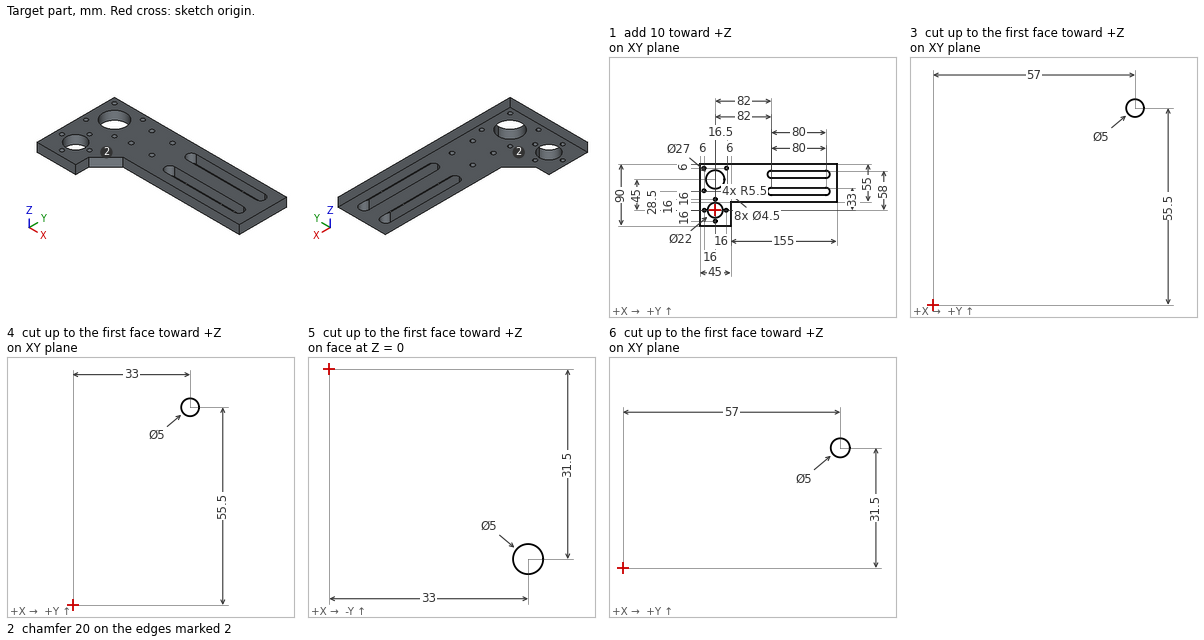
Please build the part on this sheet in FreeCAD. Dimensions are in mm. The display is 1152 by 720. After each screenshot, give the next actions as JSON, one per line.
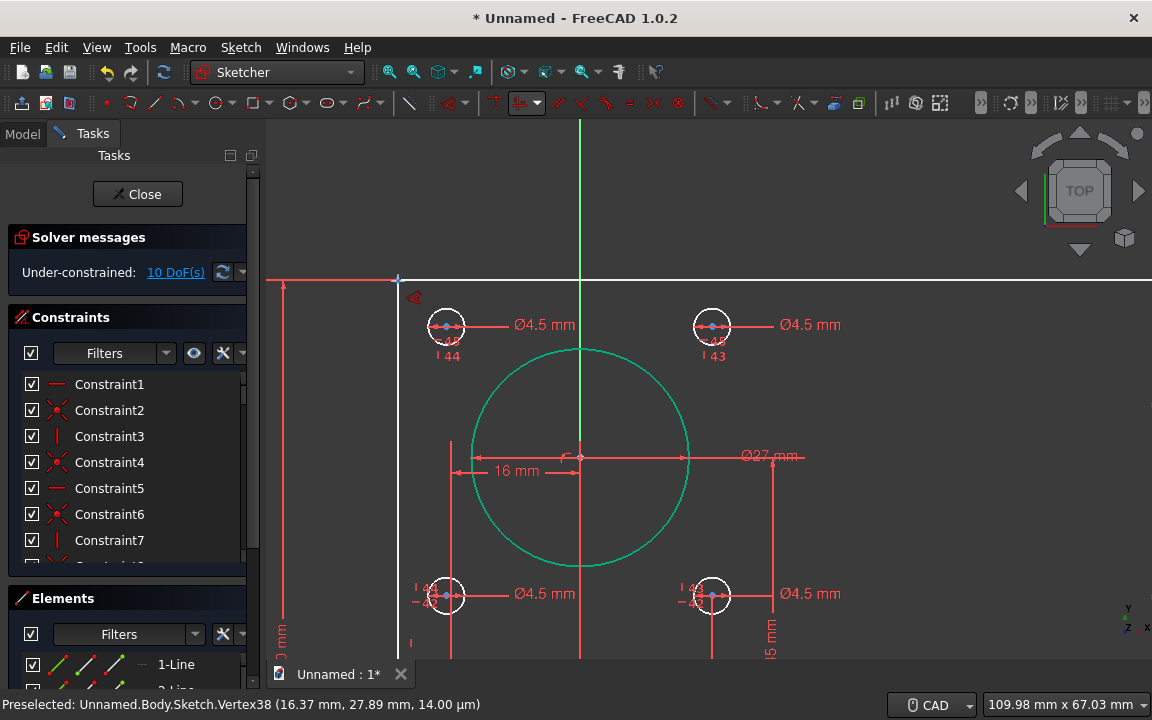
{"action": "left_click", "coordinate": [398, 280]}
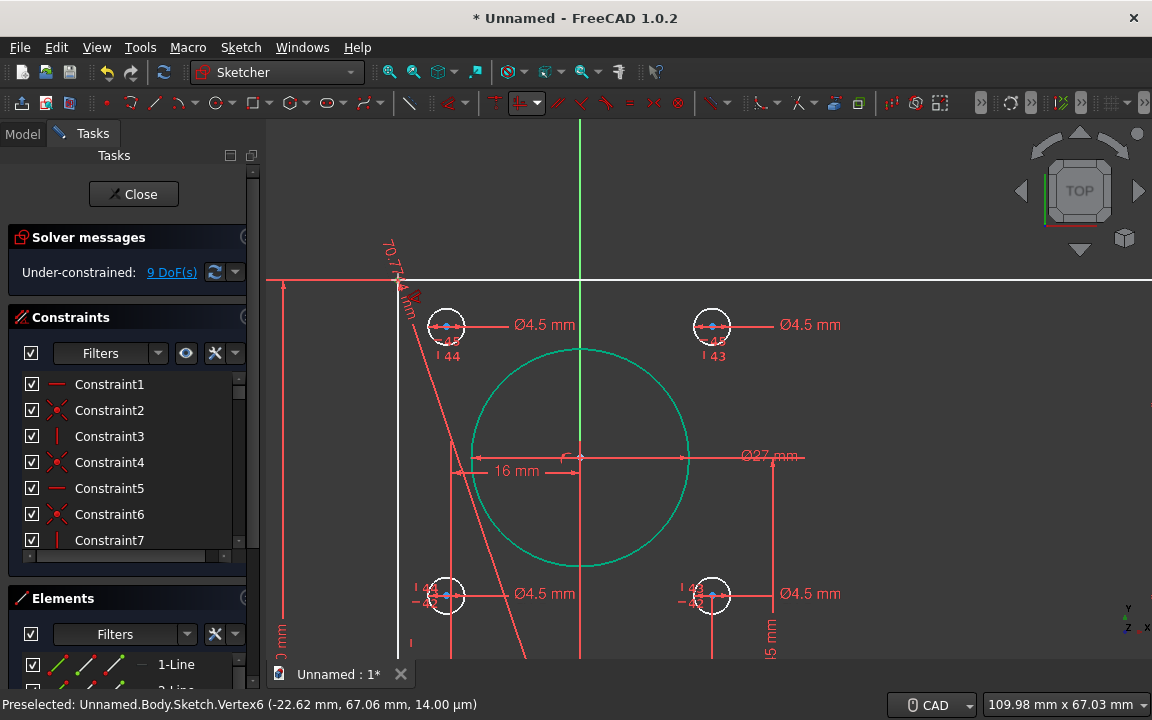
{"action": "left_click", "coordinate": [446, 596]}
{"action": "left_click", "coordinate": [422, 246]}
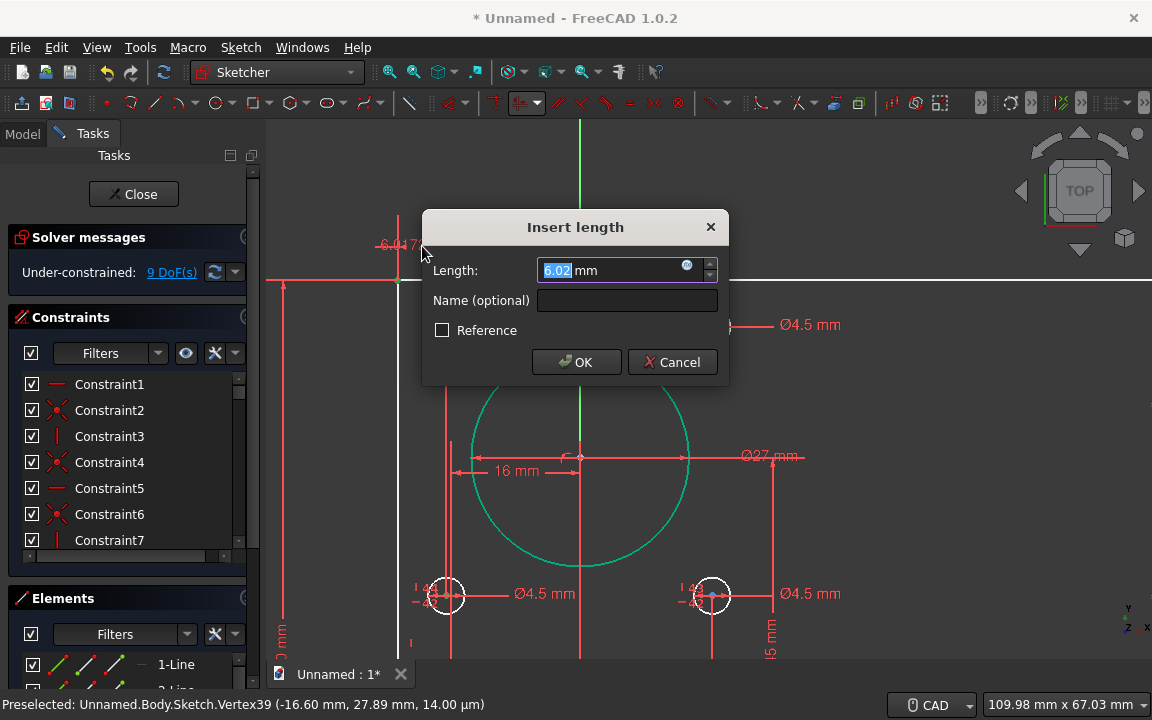
{"action": "type", "text": "6"}
{"action": "key", "text": "Return"}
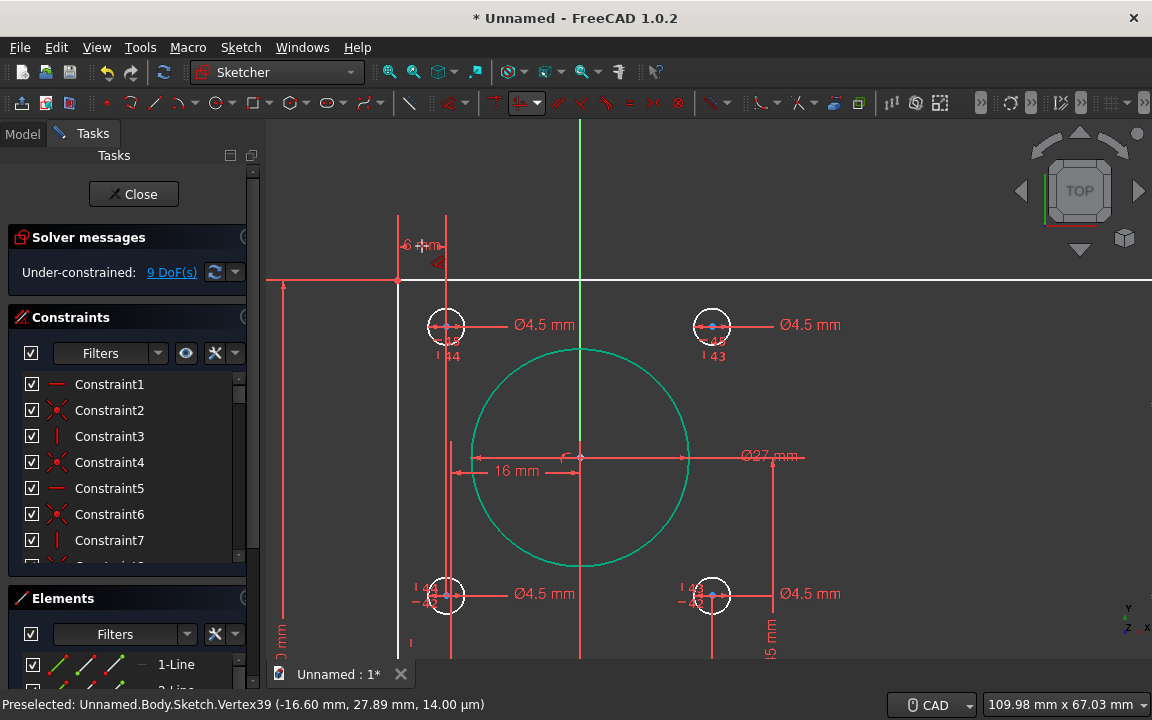
{"action": "left_click", "coordinate": [398, 280]}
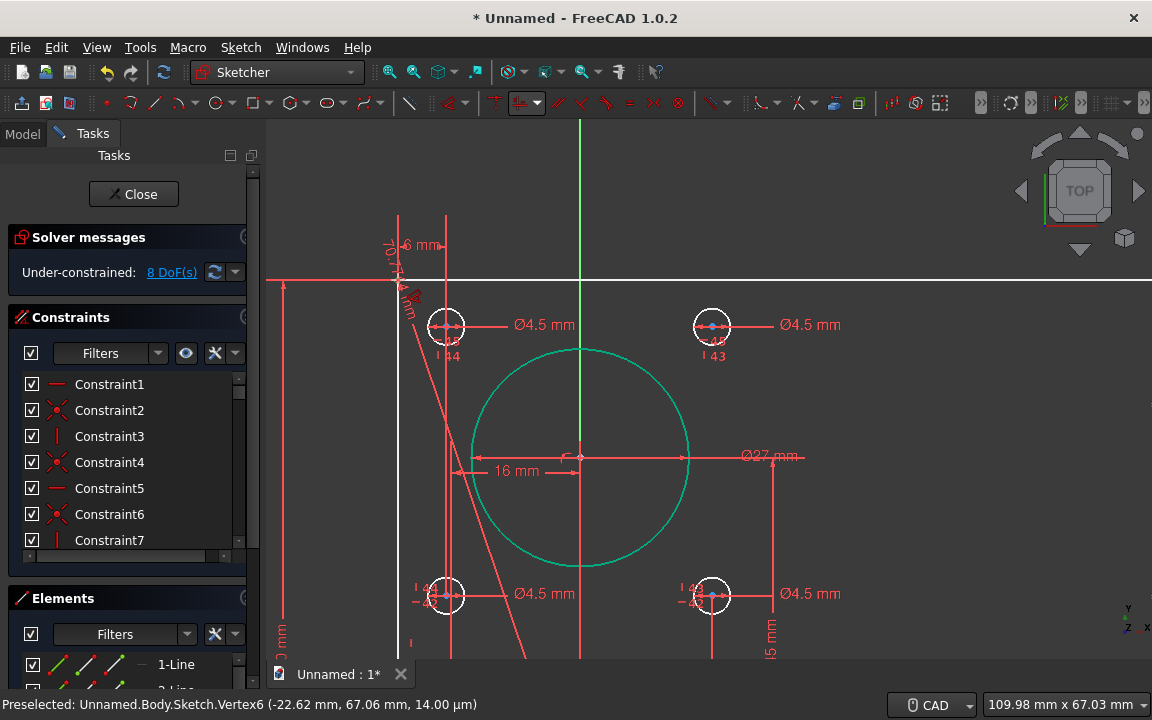
{"action": "left_click", "coordinate": [712, 327]}
{"action": "left_click", "coordinate": [364, 303]}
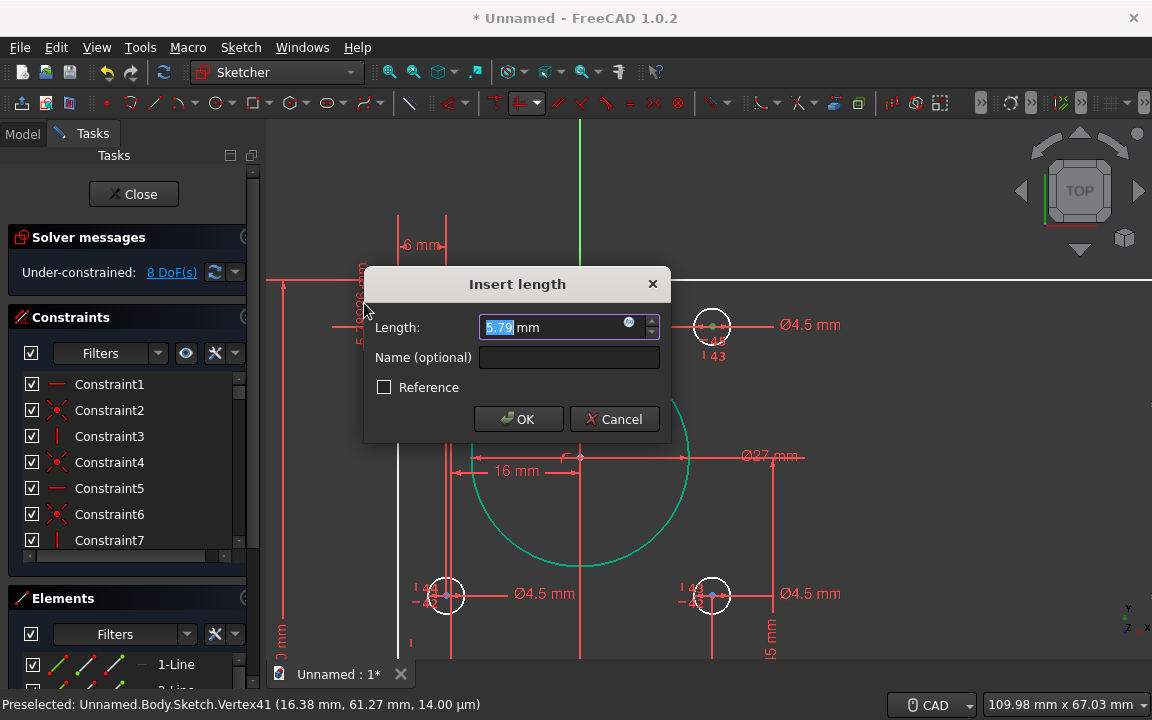
{"action": "type", "text": "6"}
{"action": "key", "text": "Return"}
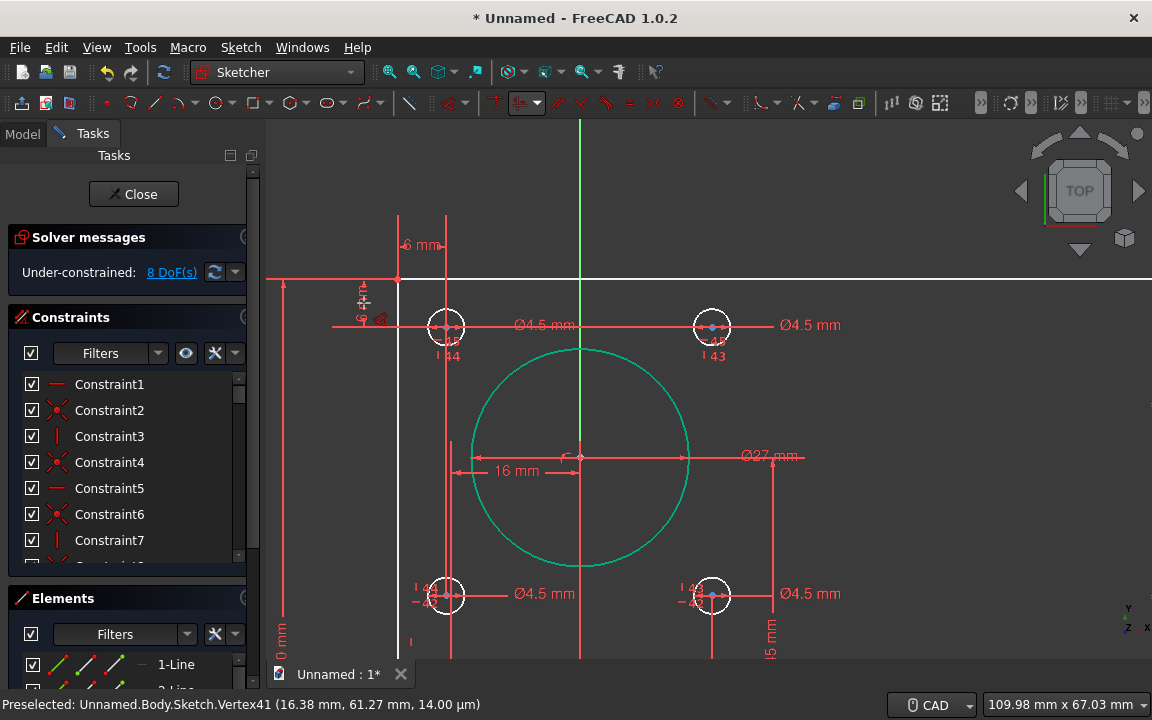
{"action": "scroll", "coordinate": [397, 281], "scroll_direction": "down", "scroll_amount": 6}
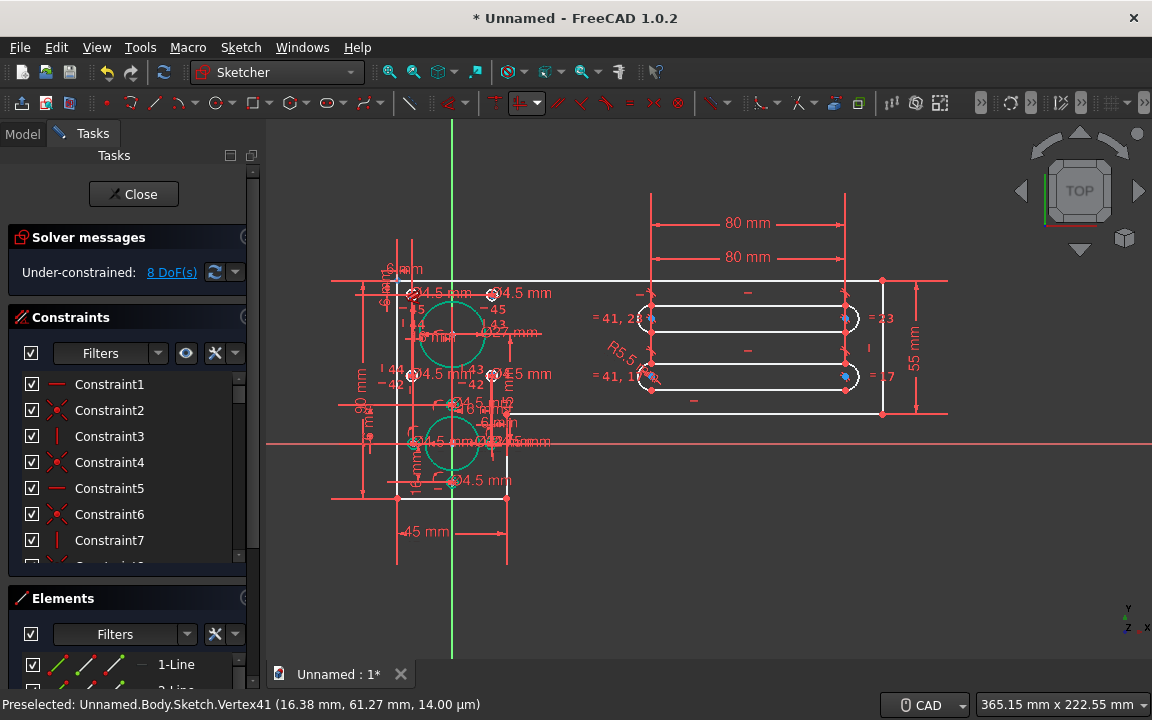
{"action": "left_click", "coordinate": [619, 414]}
{"action": "left_click", "coordinate": [695, 472]}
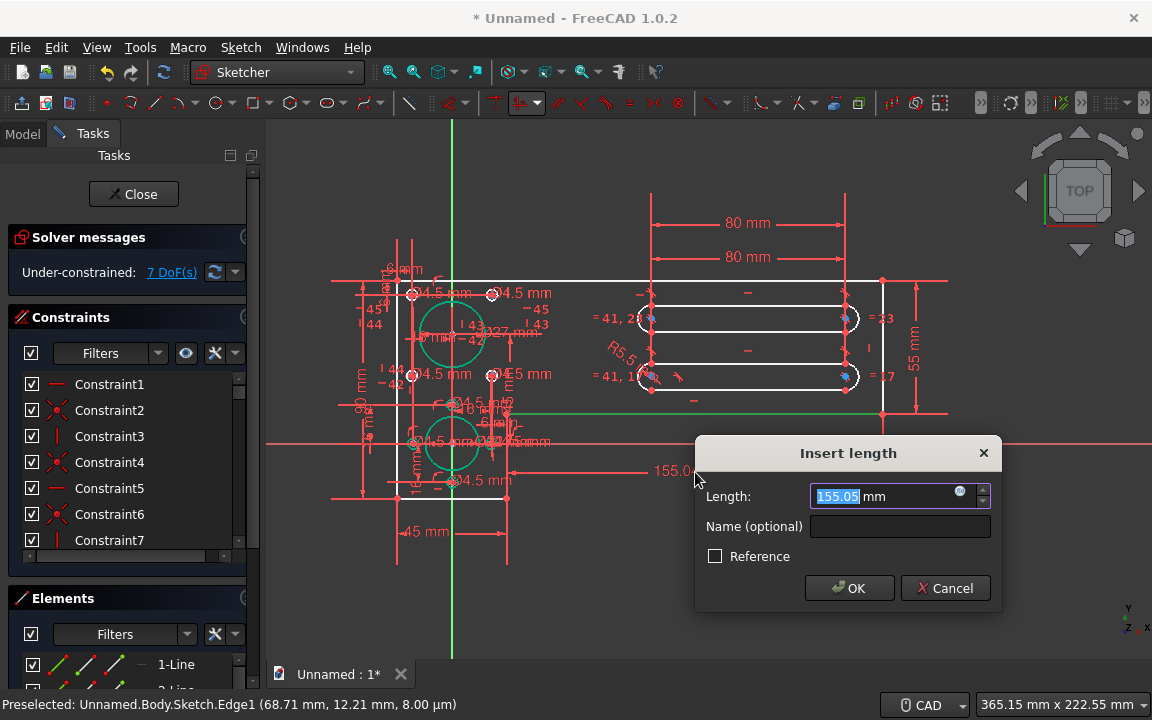
{"action": "type", "text": "155"}
{"action": "key", "text": "Return"}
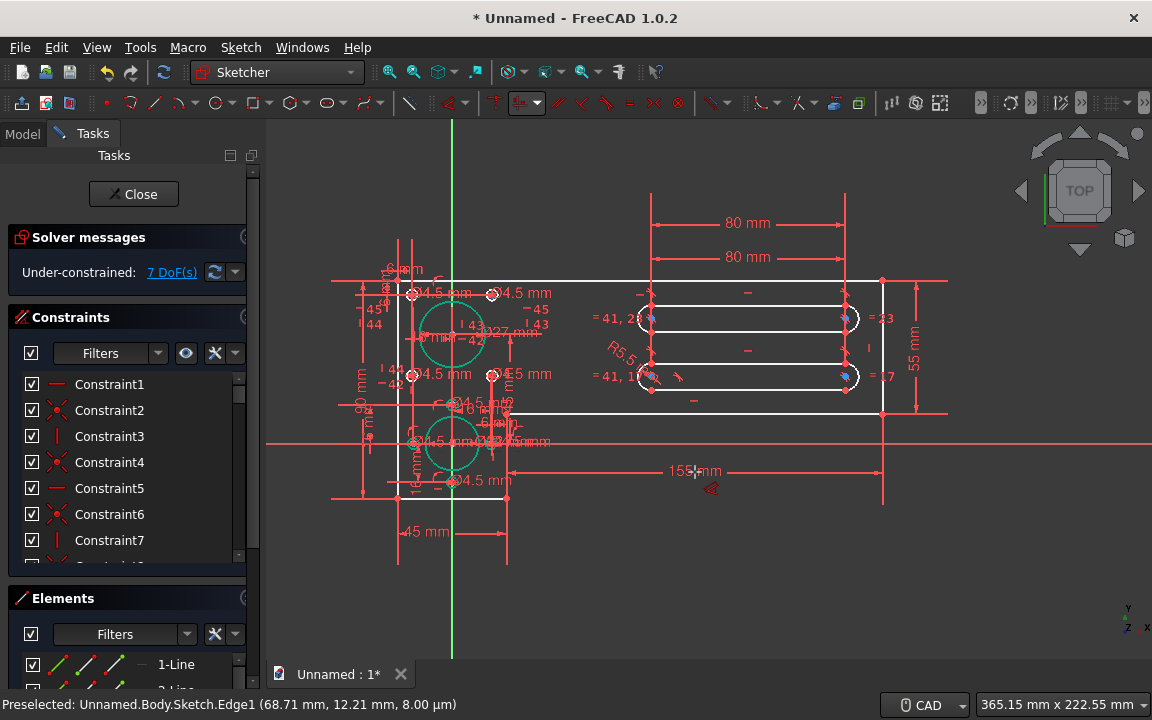
{"action": "left_click", "coordinate": [651, 364]}
{"action": "left_click", "coordinate": [552, 478]}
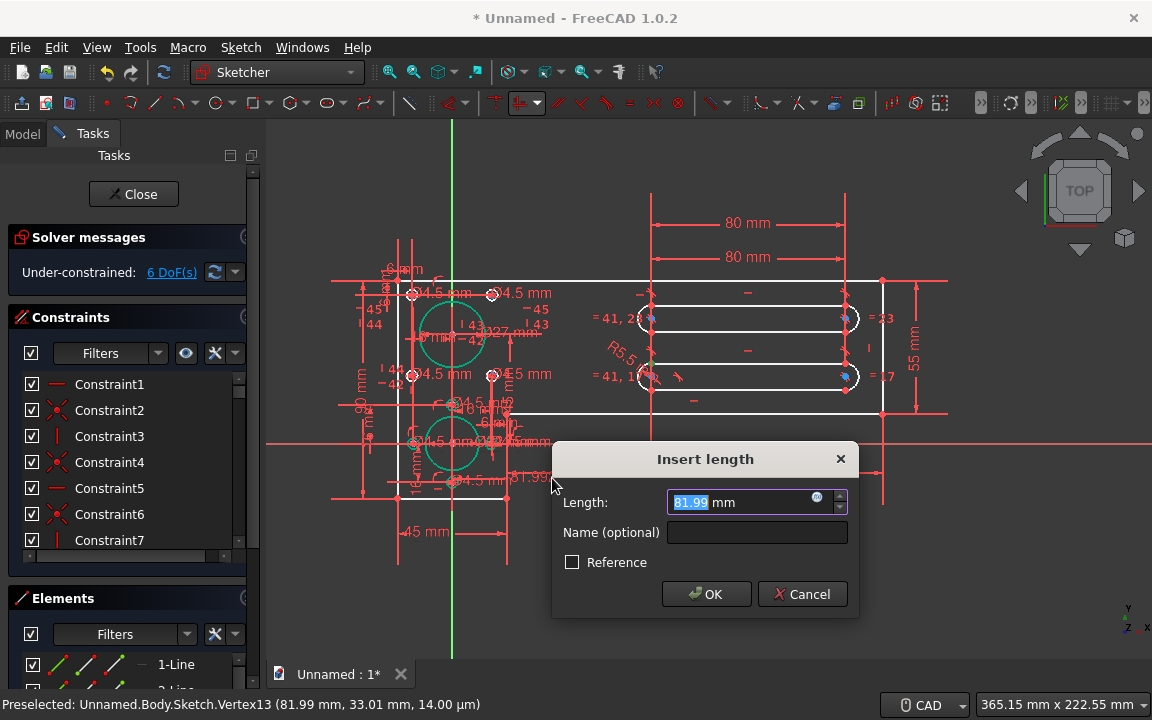
{"action": "type", "text": "82"}
{"action": "key", "text": "Return"}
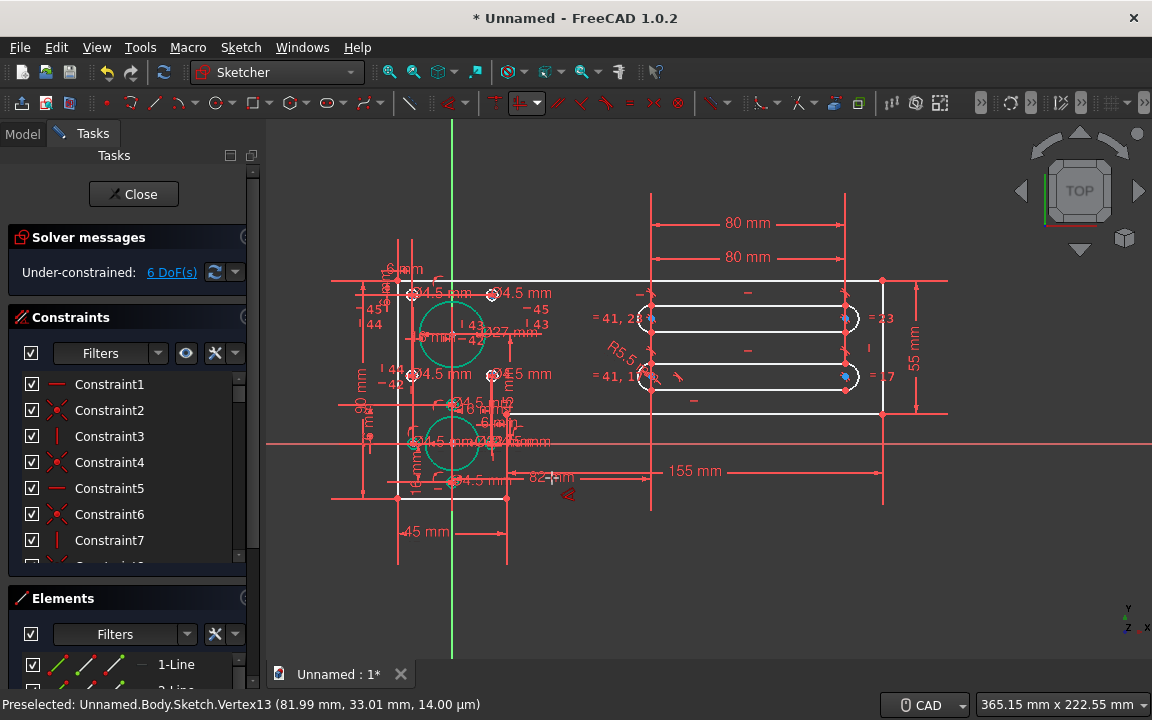
{"action": "left_click", "coordinate": [651, 364]}
{"action": "left_click", "coordinate": [298, 422]}